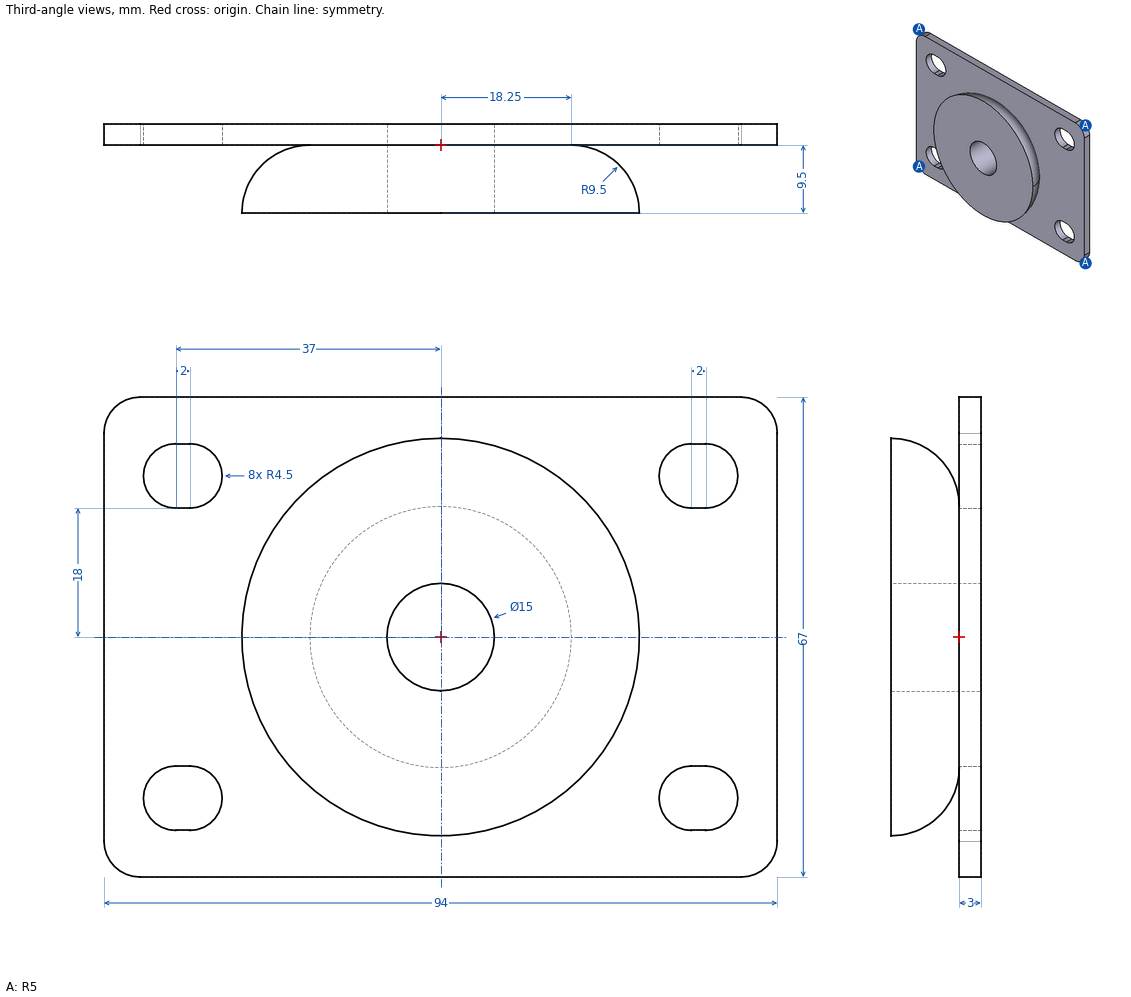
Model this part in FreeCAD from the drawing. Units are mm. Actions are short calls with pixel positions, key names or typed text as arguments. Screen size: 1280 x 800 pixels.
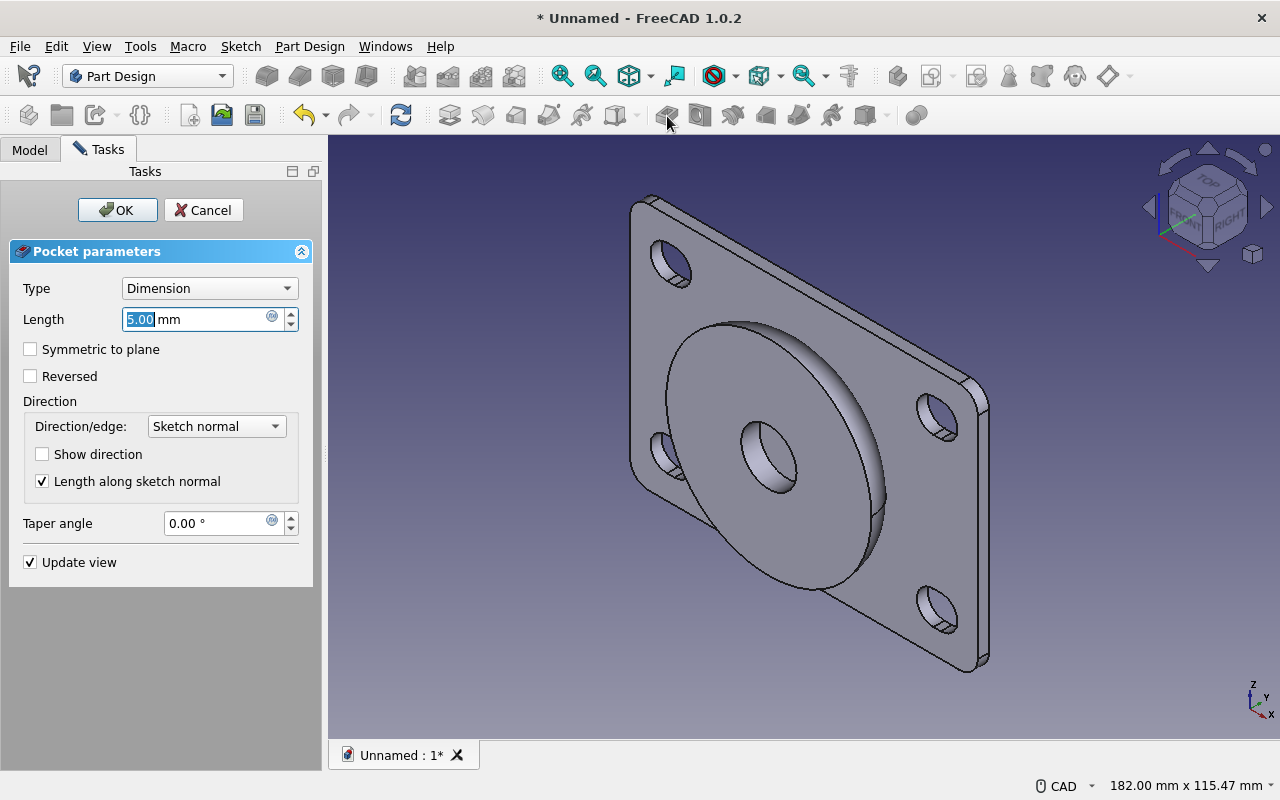
click(210, 288)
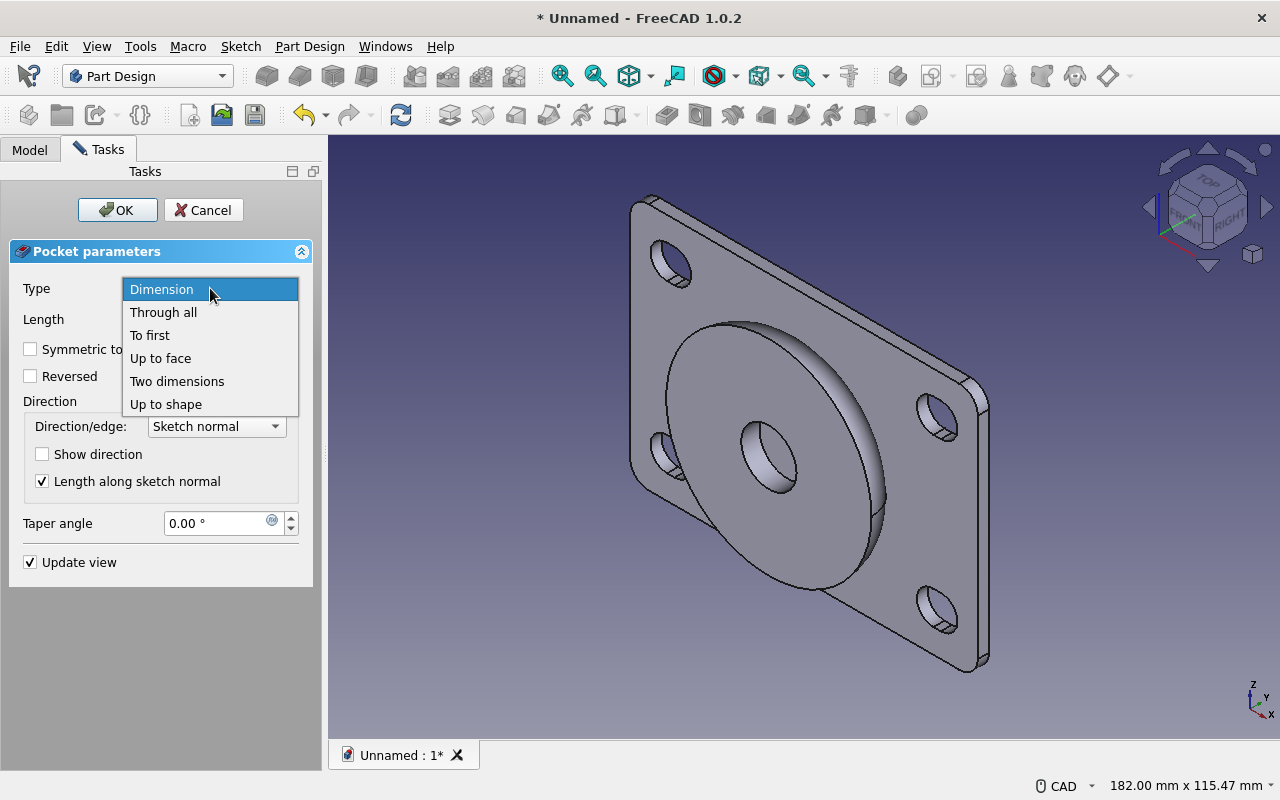
click(208, 312)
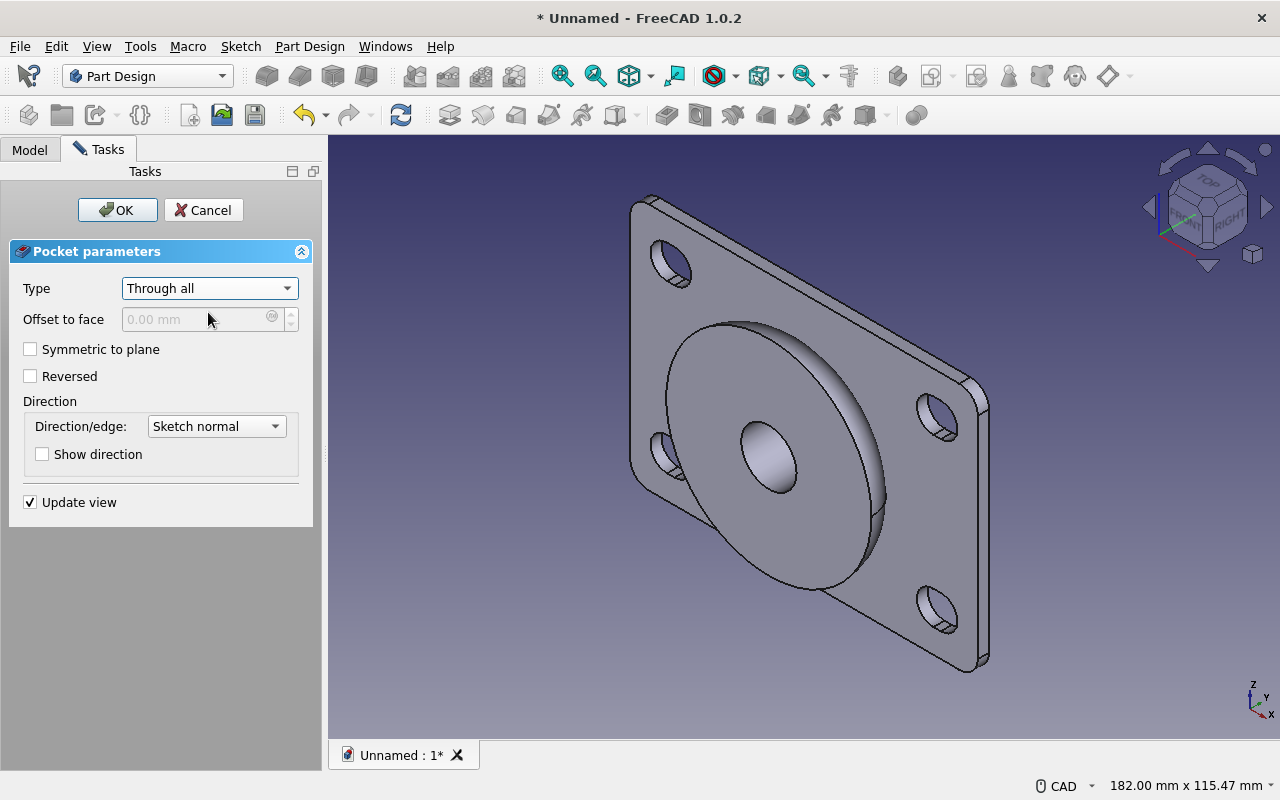
click(118, 210)